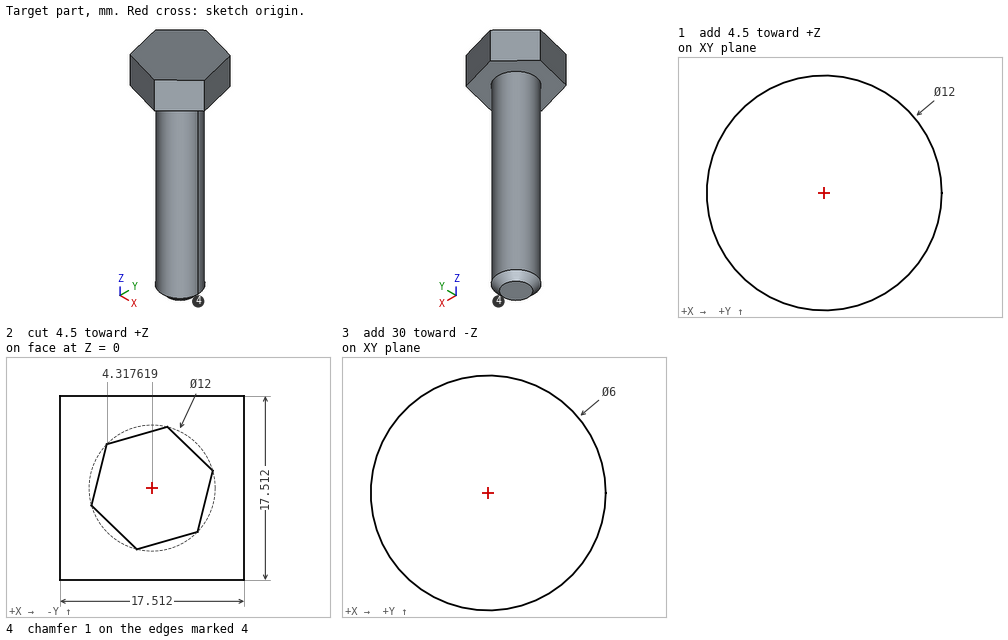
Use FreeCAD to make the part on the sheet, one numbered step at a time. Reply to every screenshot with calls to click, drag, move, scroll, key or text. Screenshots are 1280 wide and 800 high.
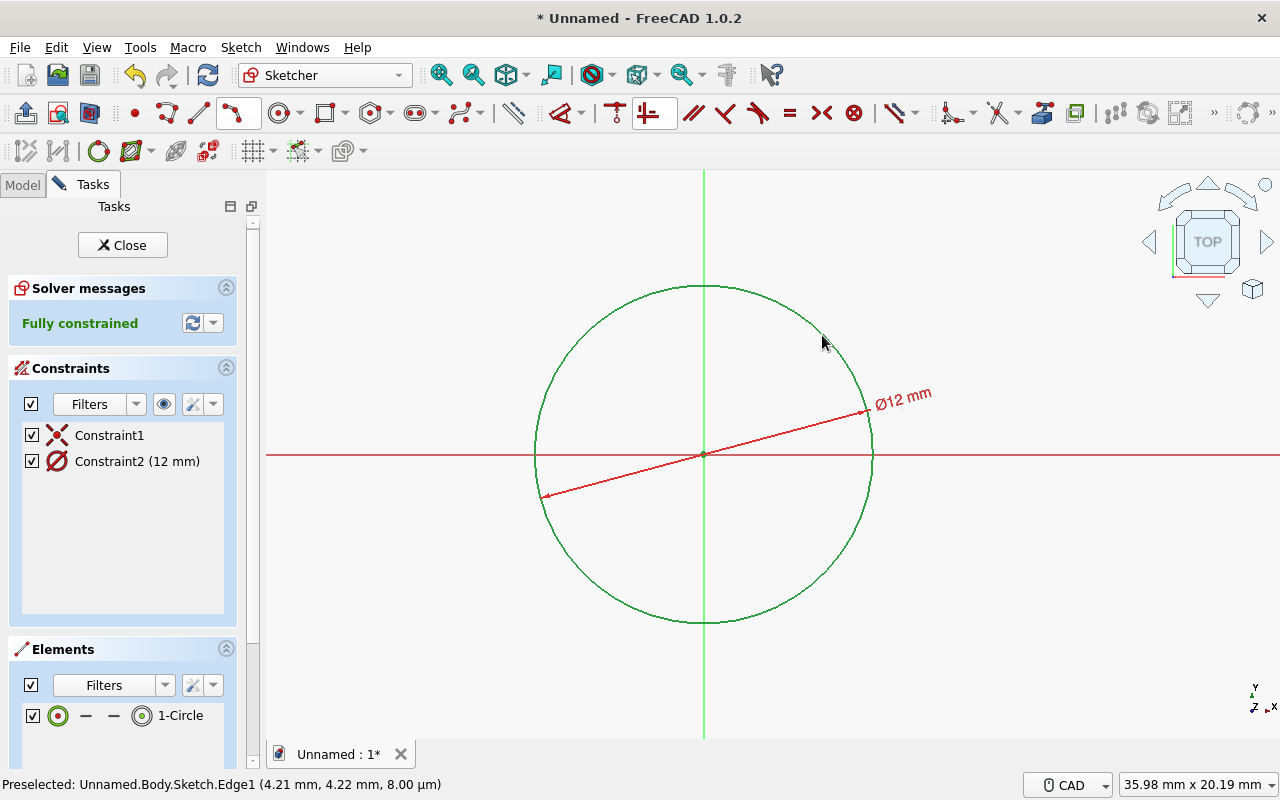
click(123, 245)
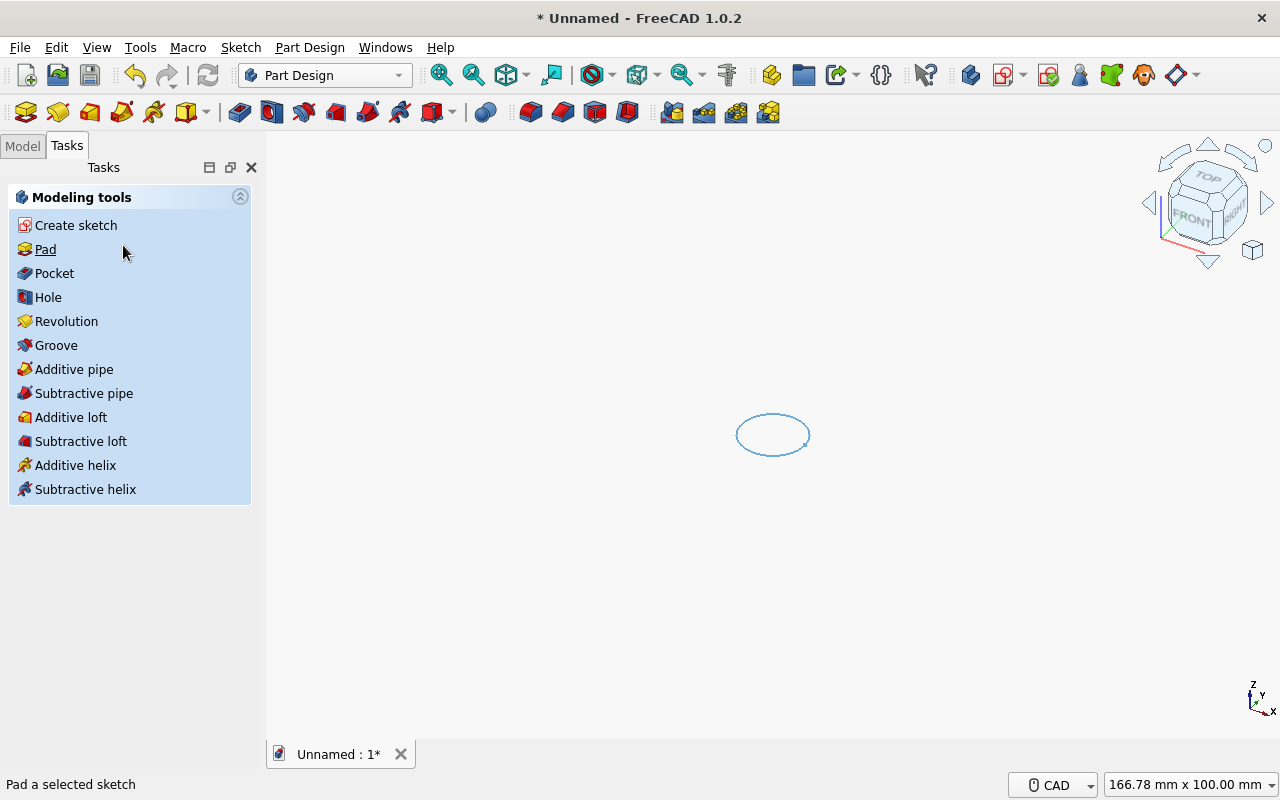
click(26, 112)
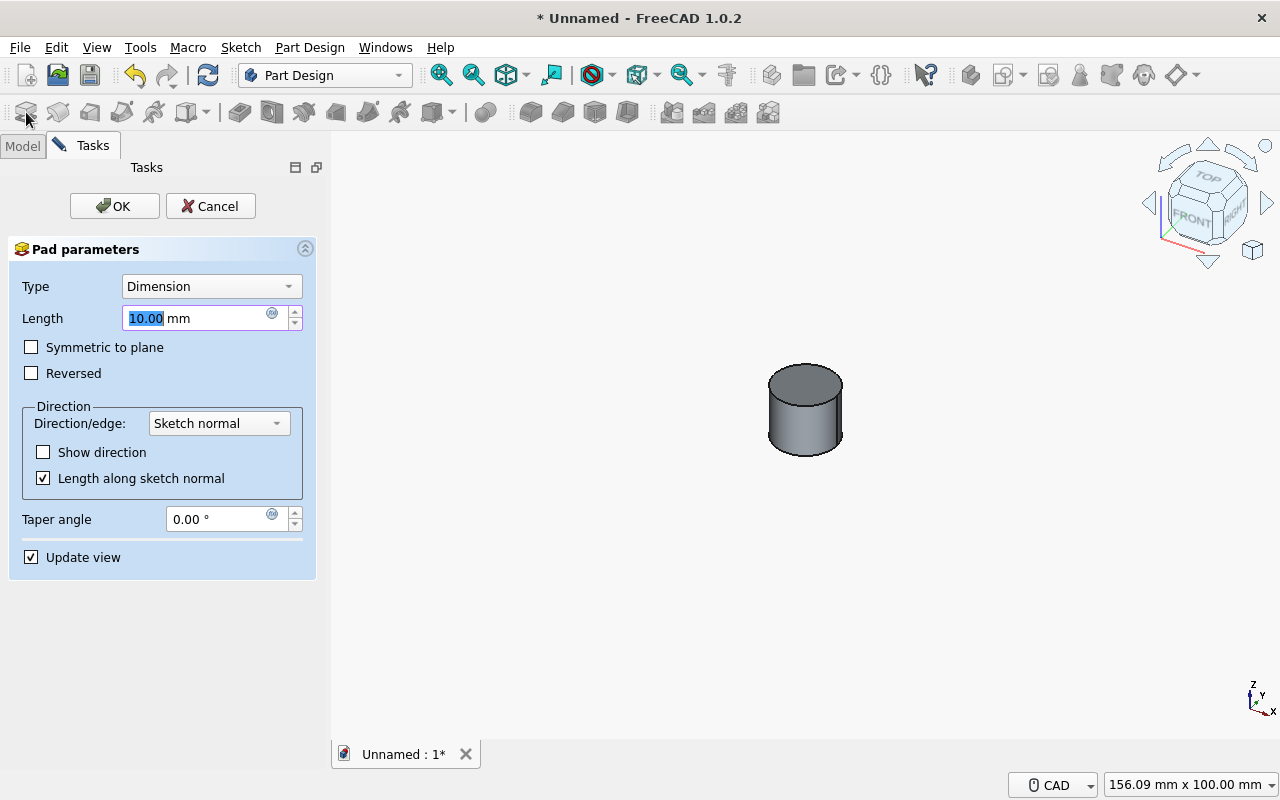
text(4.5)
key(Tab)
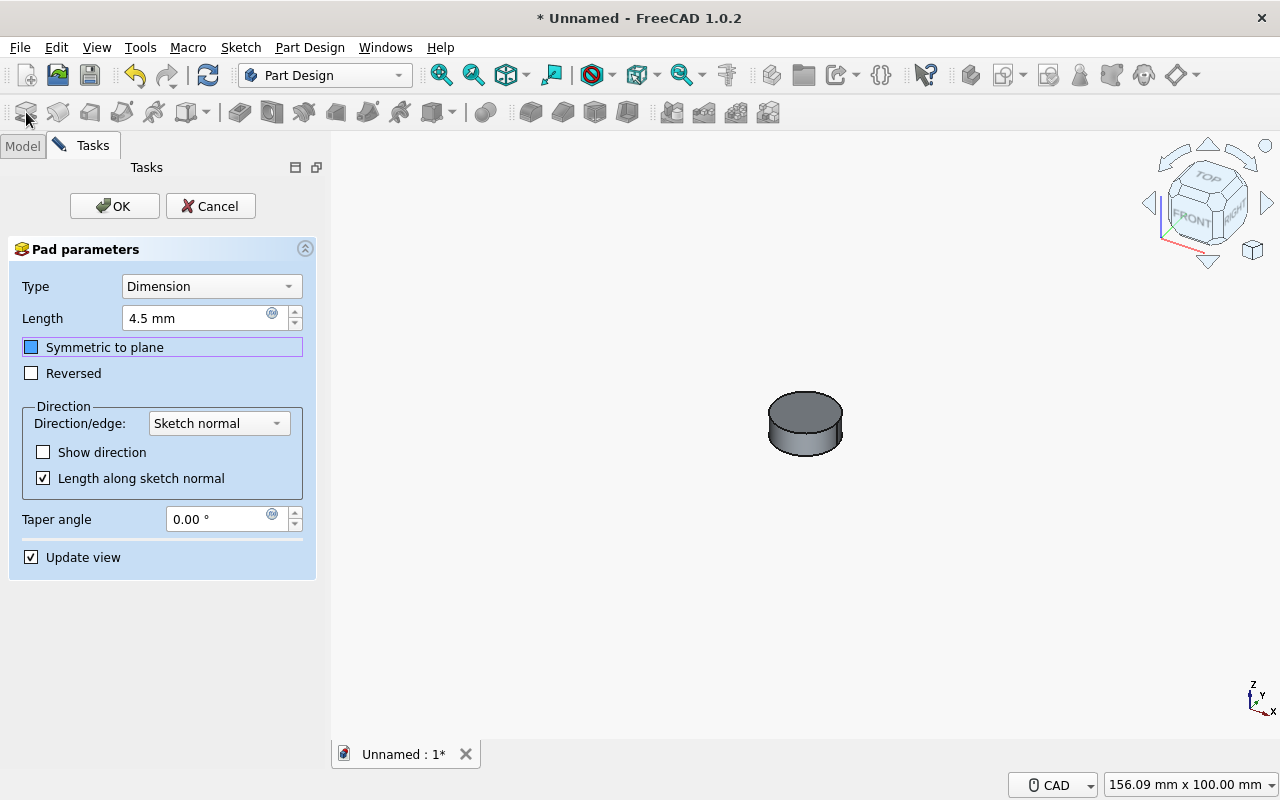
click(115, 206)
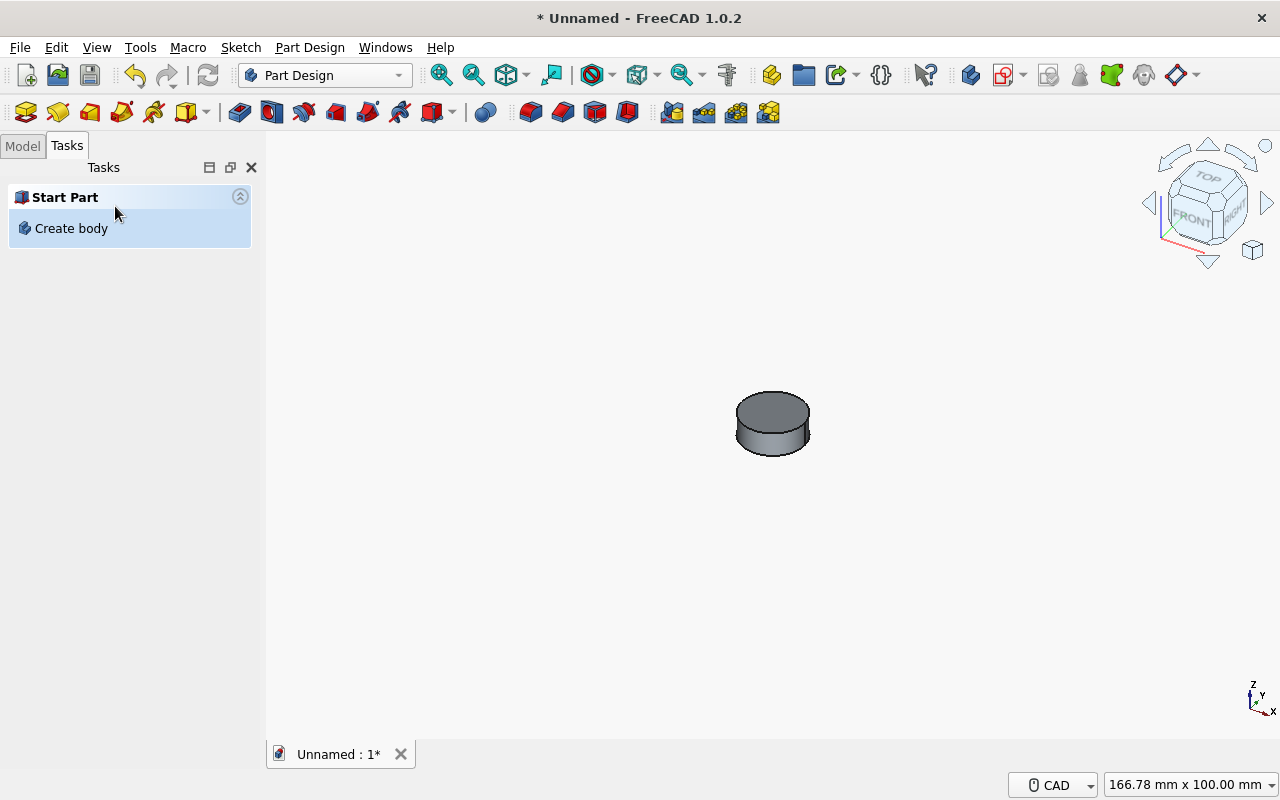
click(442, 76)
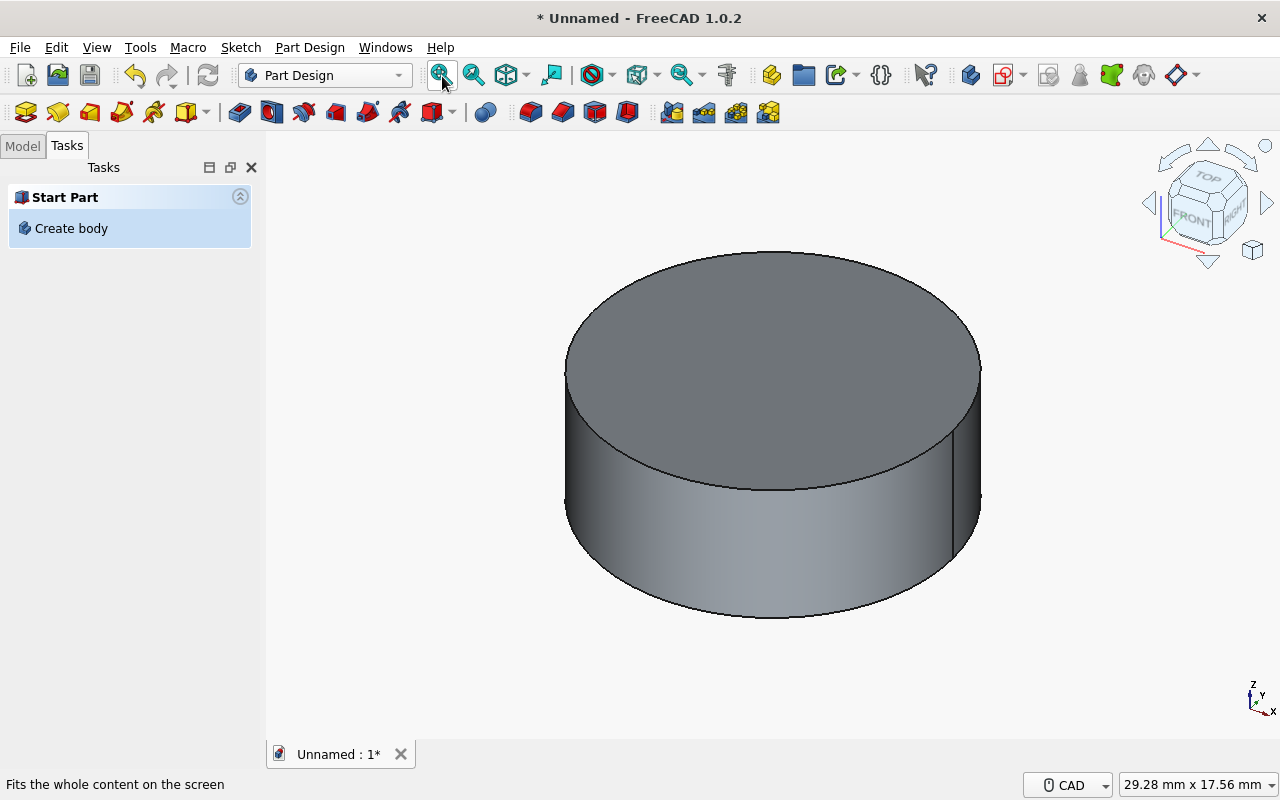
key(5)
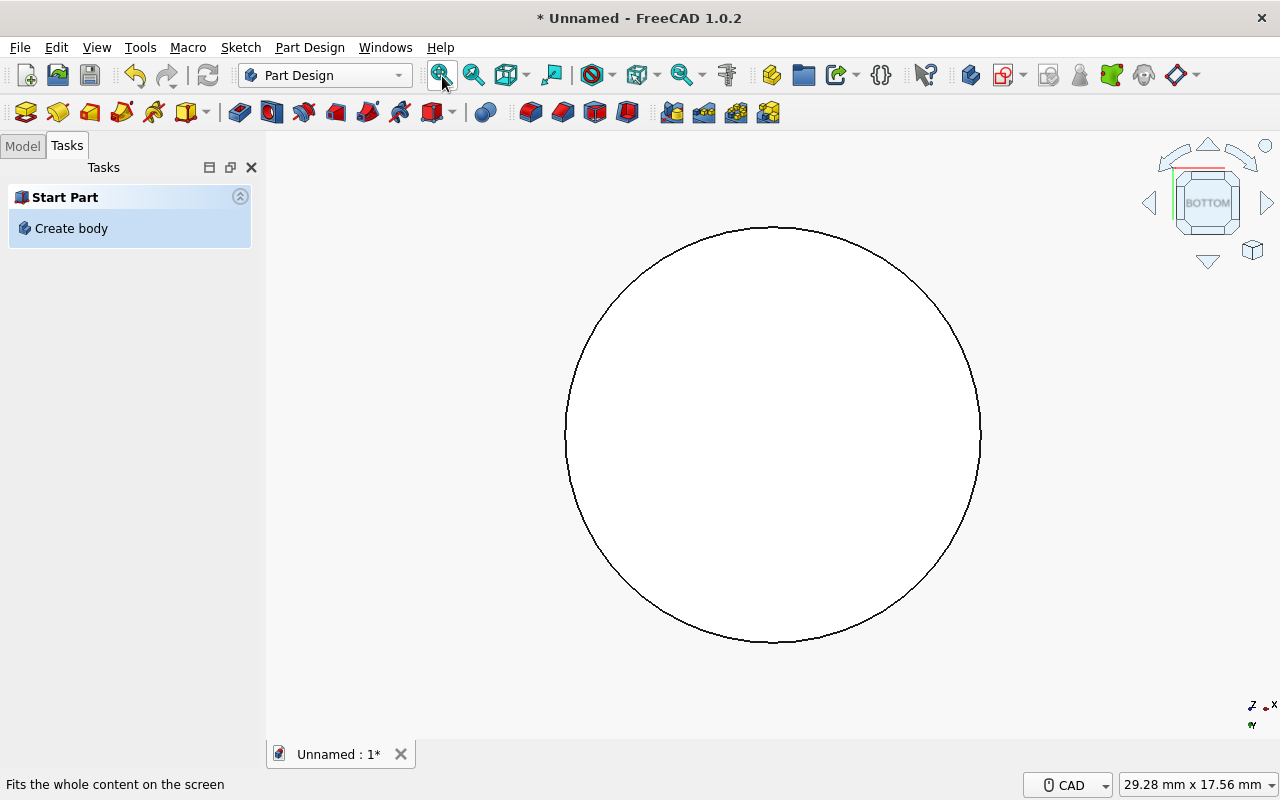
click(773, 434)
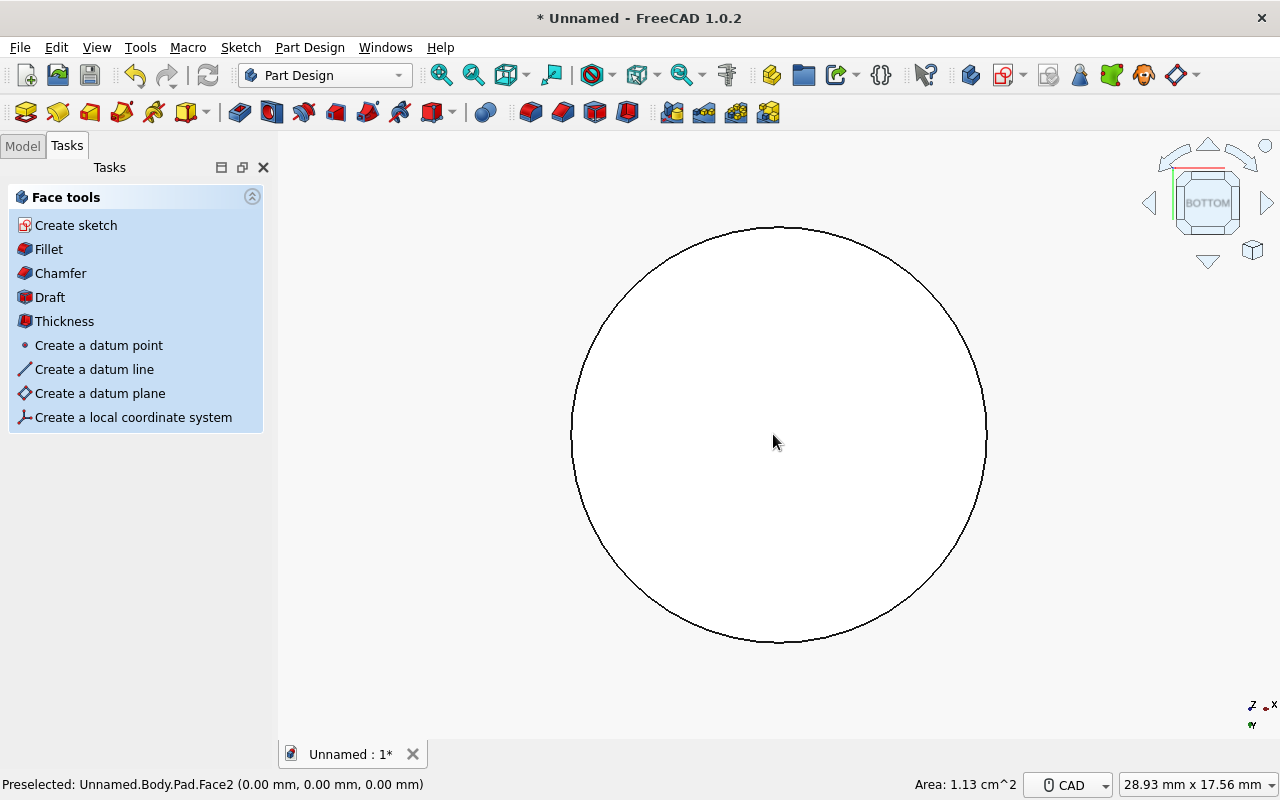
click(1004, 76)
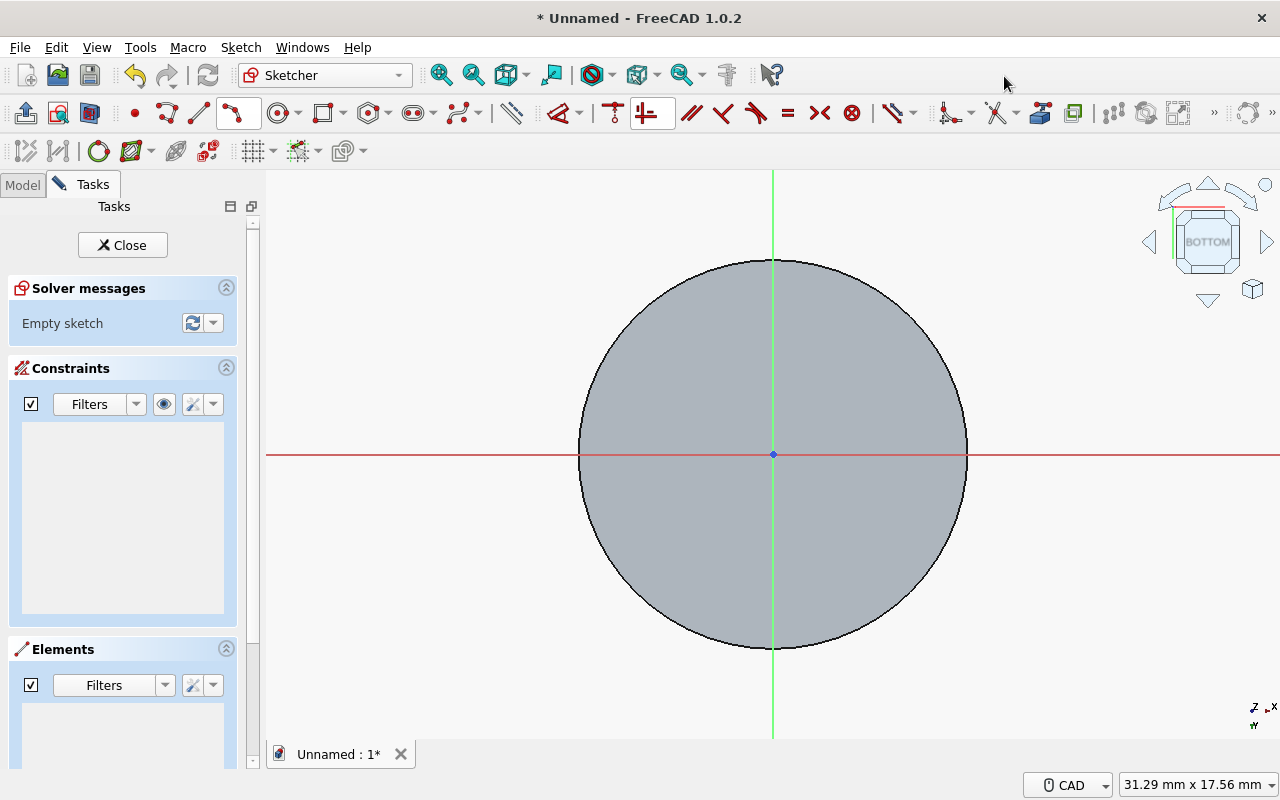
scroll(565, 455, down, 2)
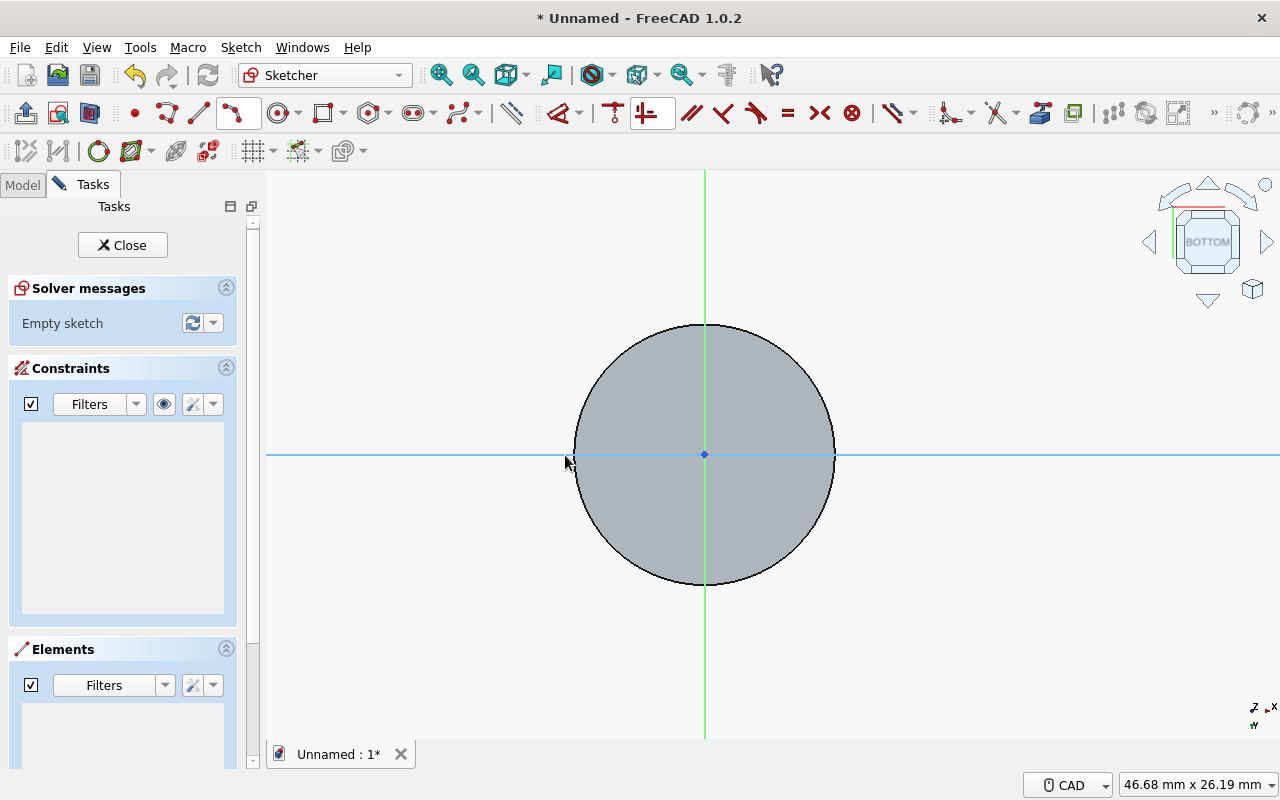
click(346, 114)